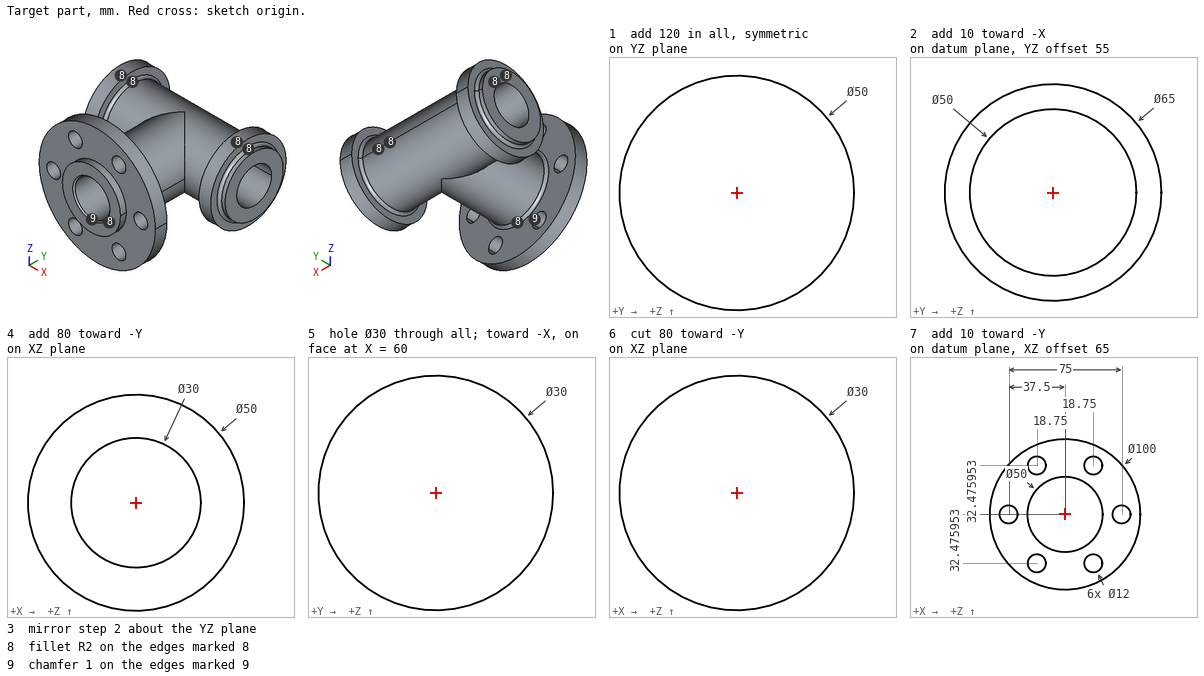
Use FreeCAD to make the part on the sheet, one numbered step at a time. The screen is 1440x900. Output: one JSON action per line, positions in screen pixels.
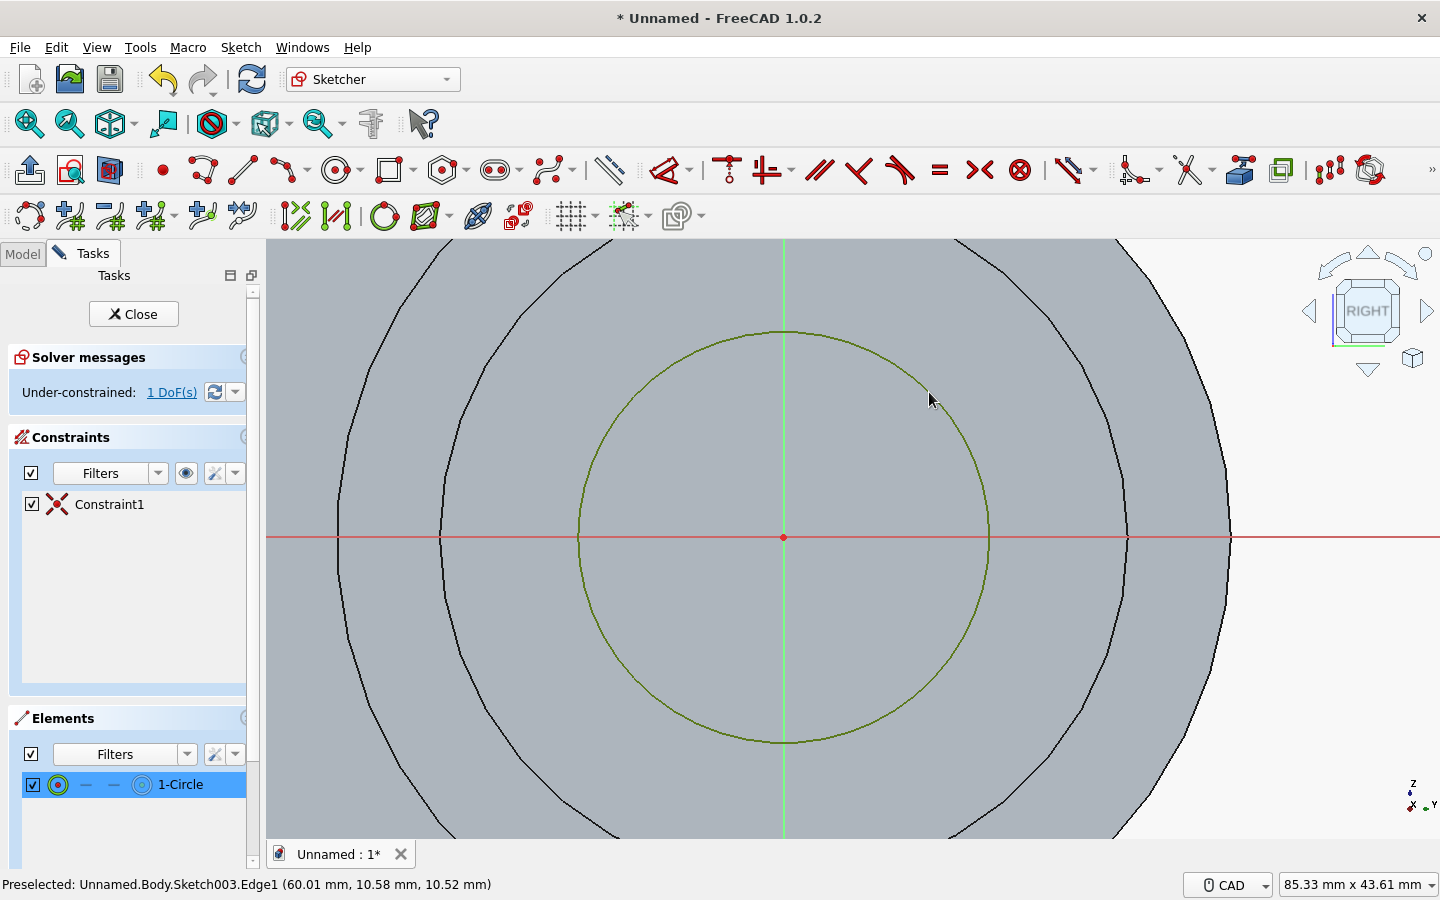
{"action": "key", "text": "k o"}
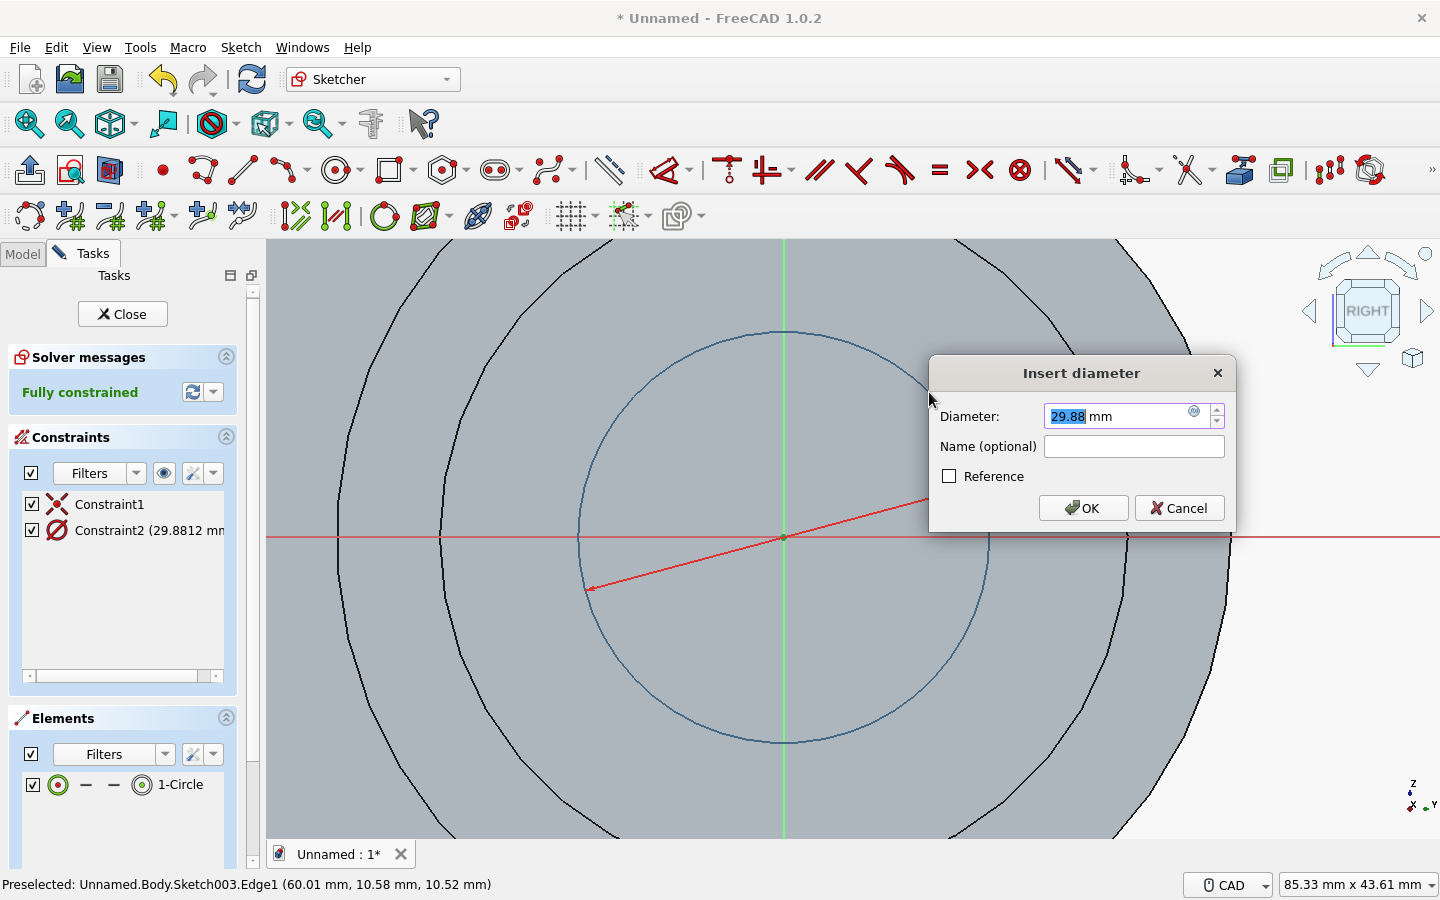
{"action": "type", "text": "30"}
{"action": "key", "text": "Return"}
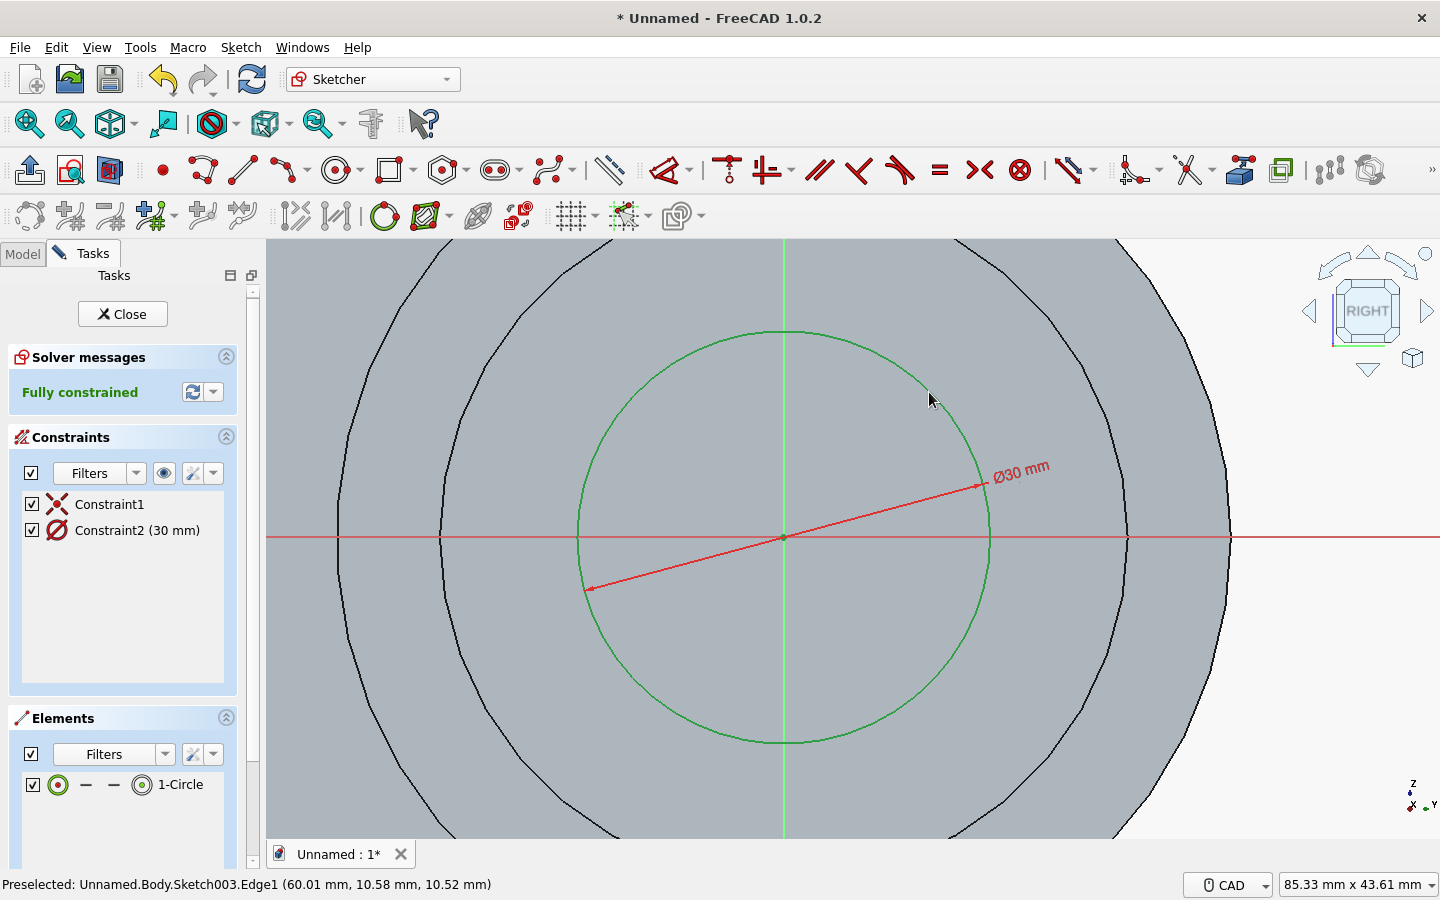
{"action": "left_click", "coordinate": [123, 314]}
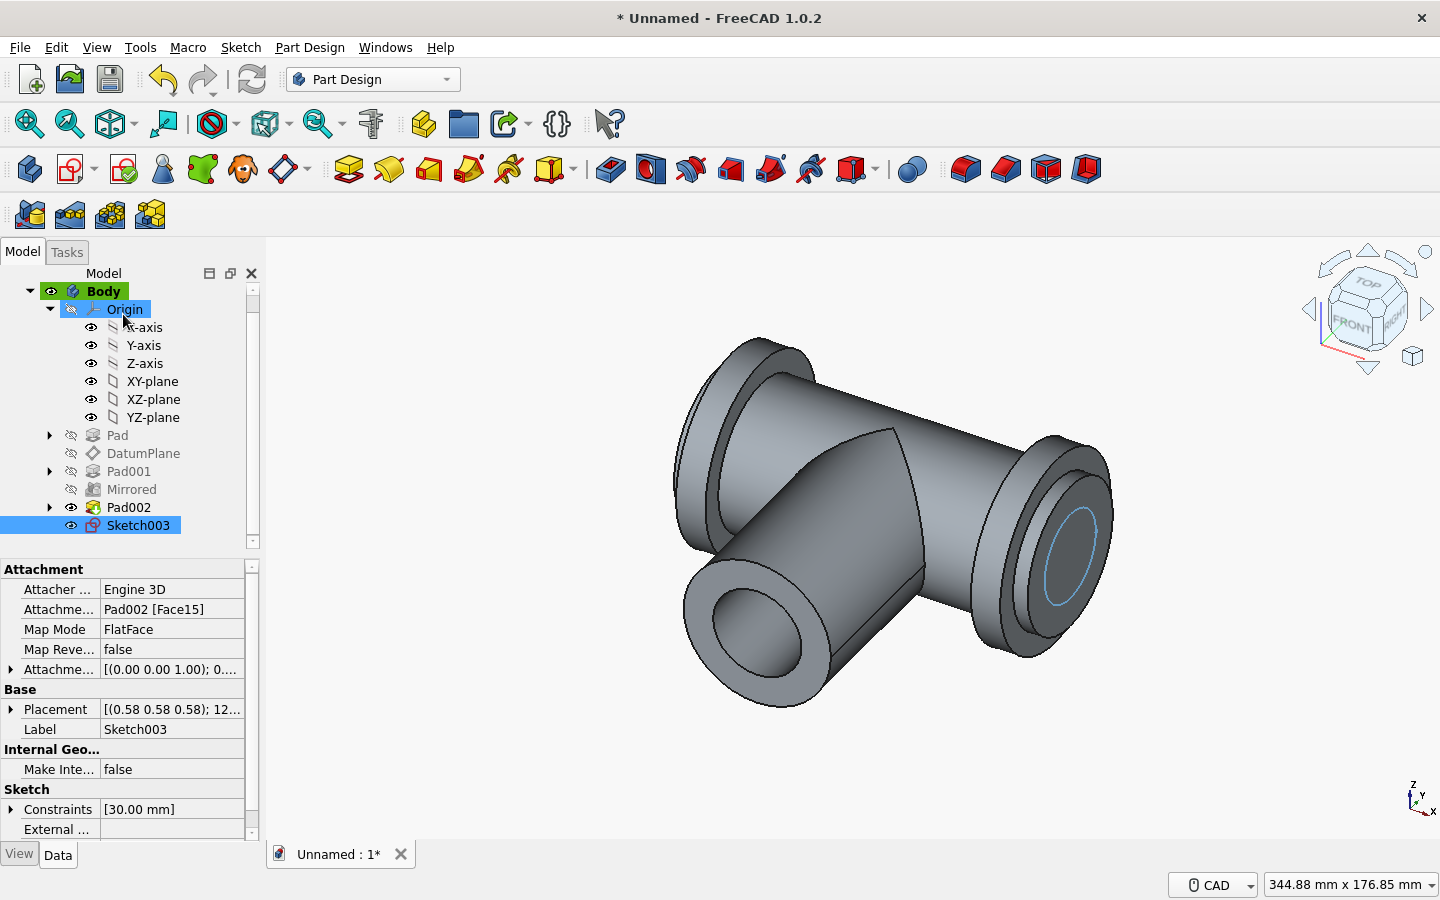
{"action": "left_click", "coordinate": [652, 170]}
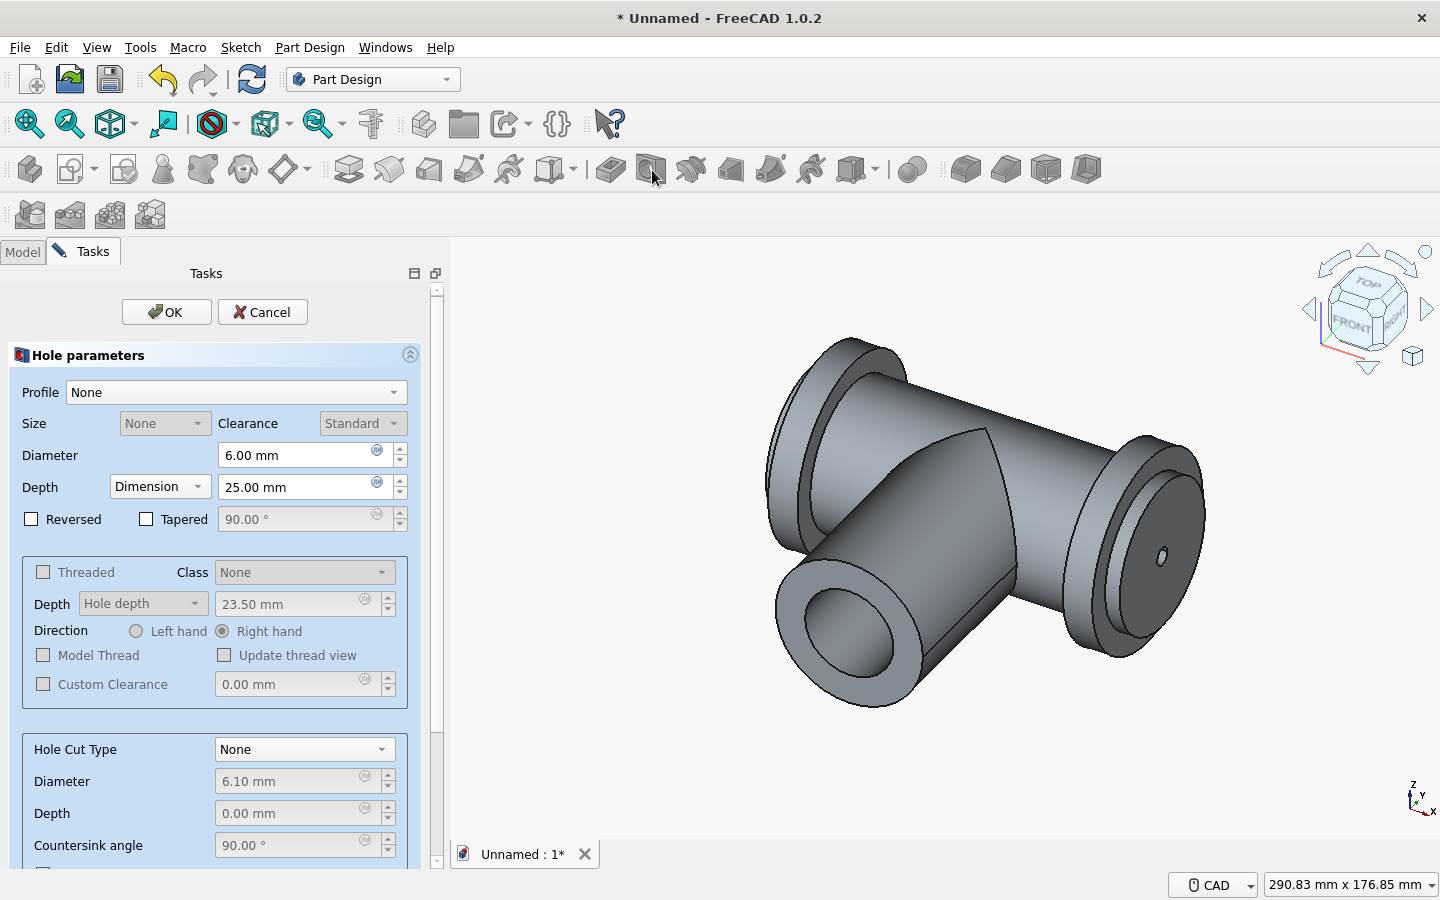
{"action": "triple_click", "coordinate": [305, 455]}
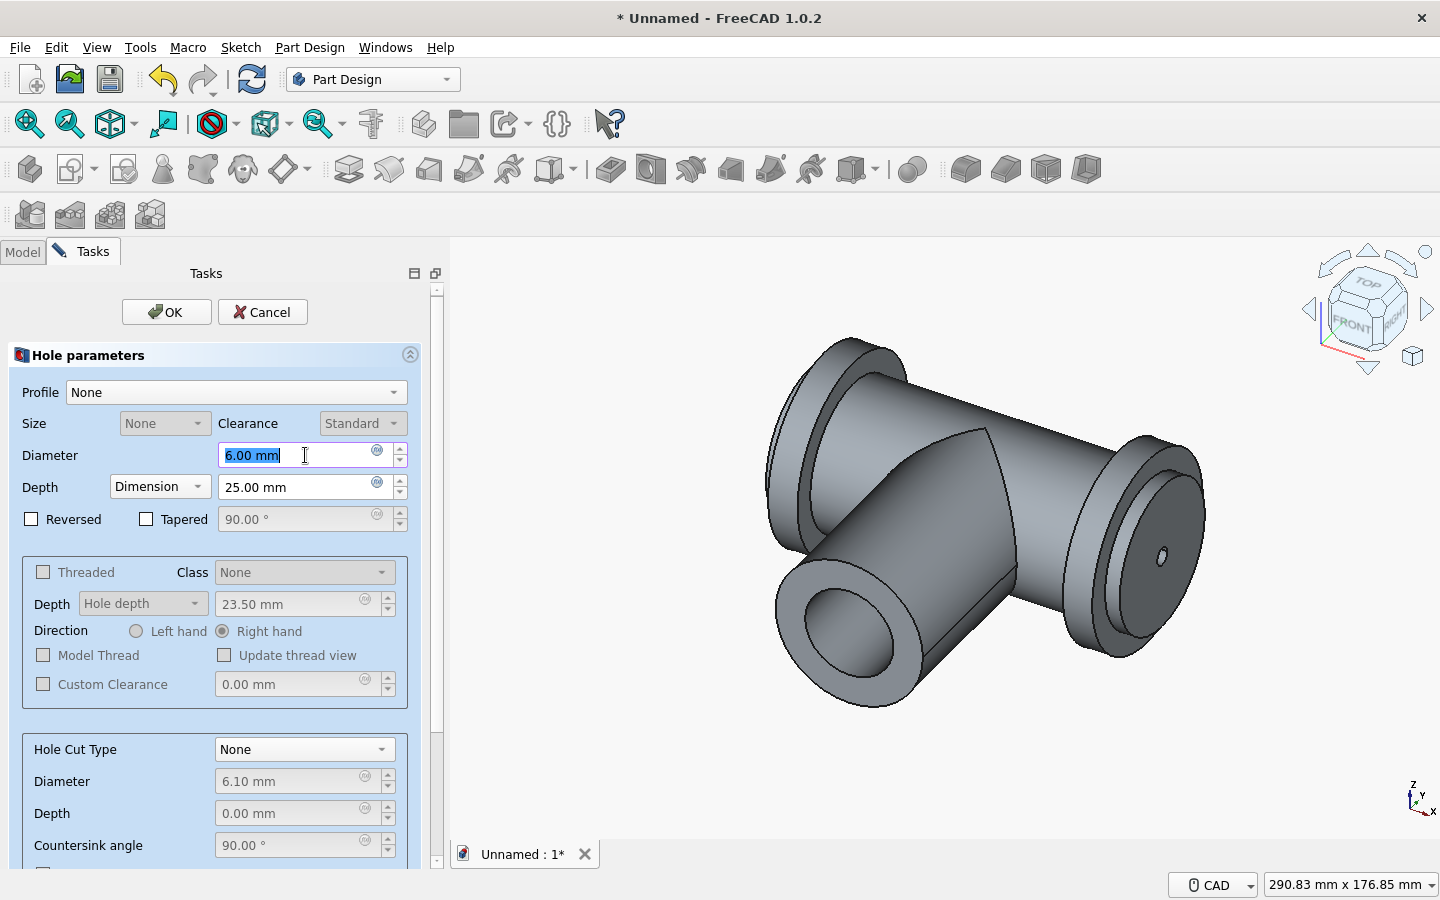
{"action": "type", "text": "30"}
{"action": "key", "text": "Tab"}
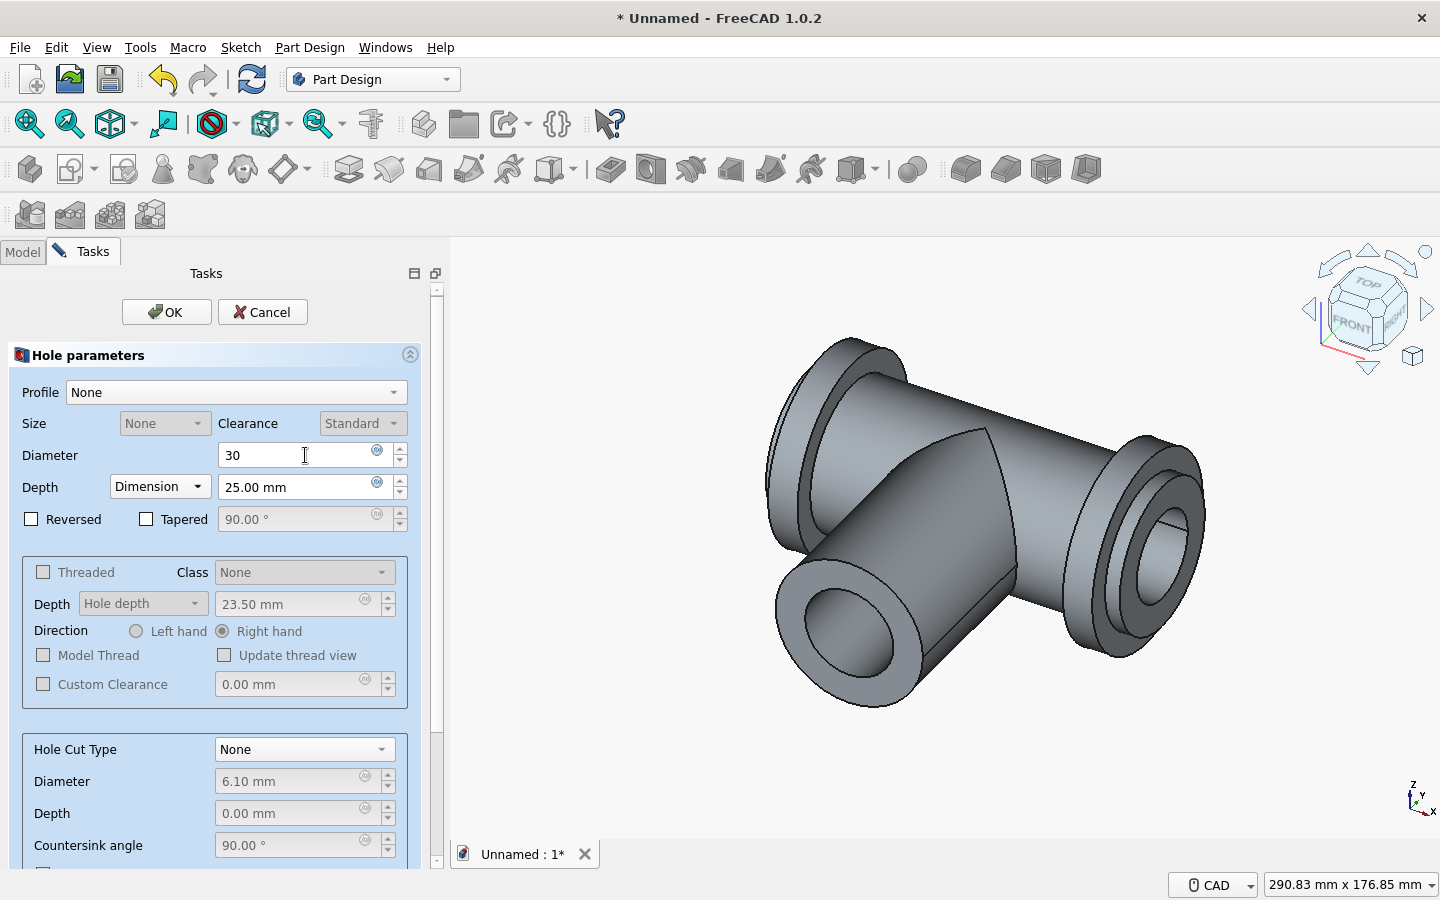
{"action": "left_click", "coordinate": [161, 486]}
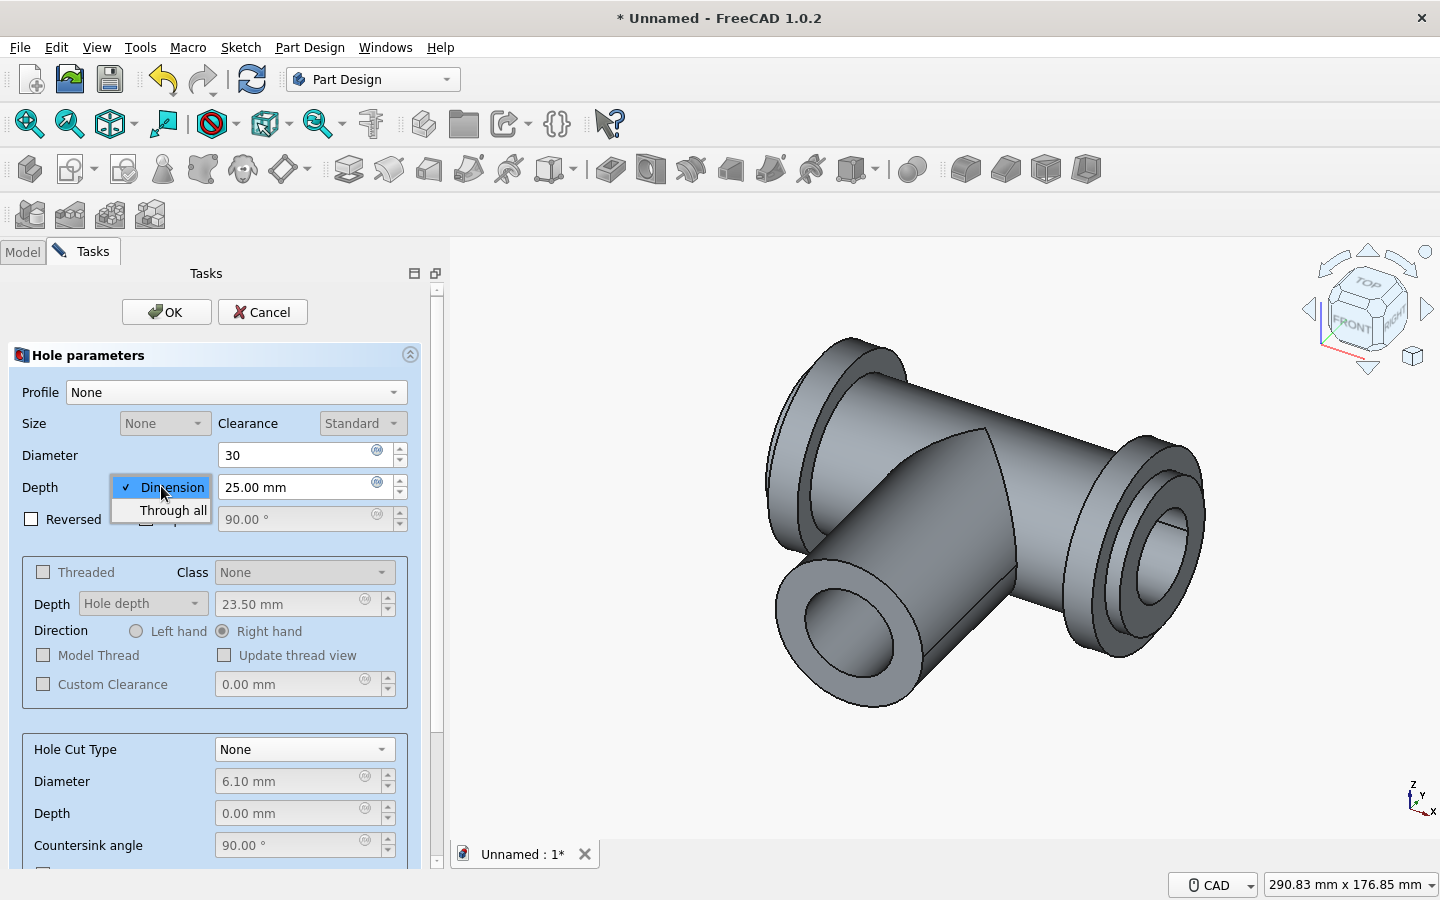
{"action": "left_click", "coordinate": [160, 510]}